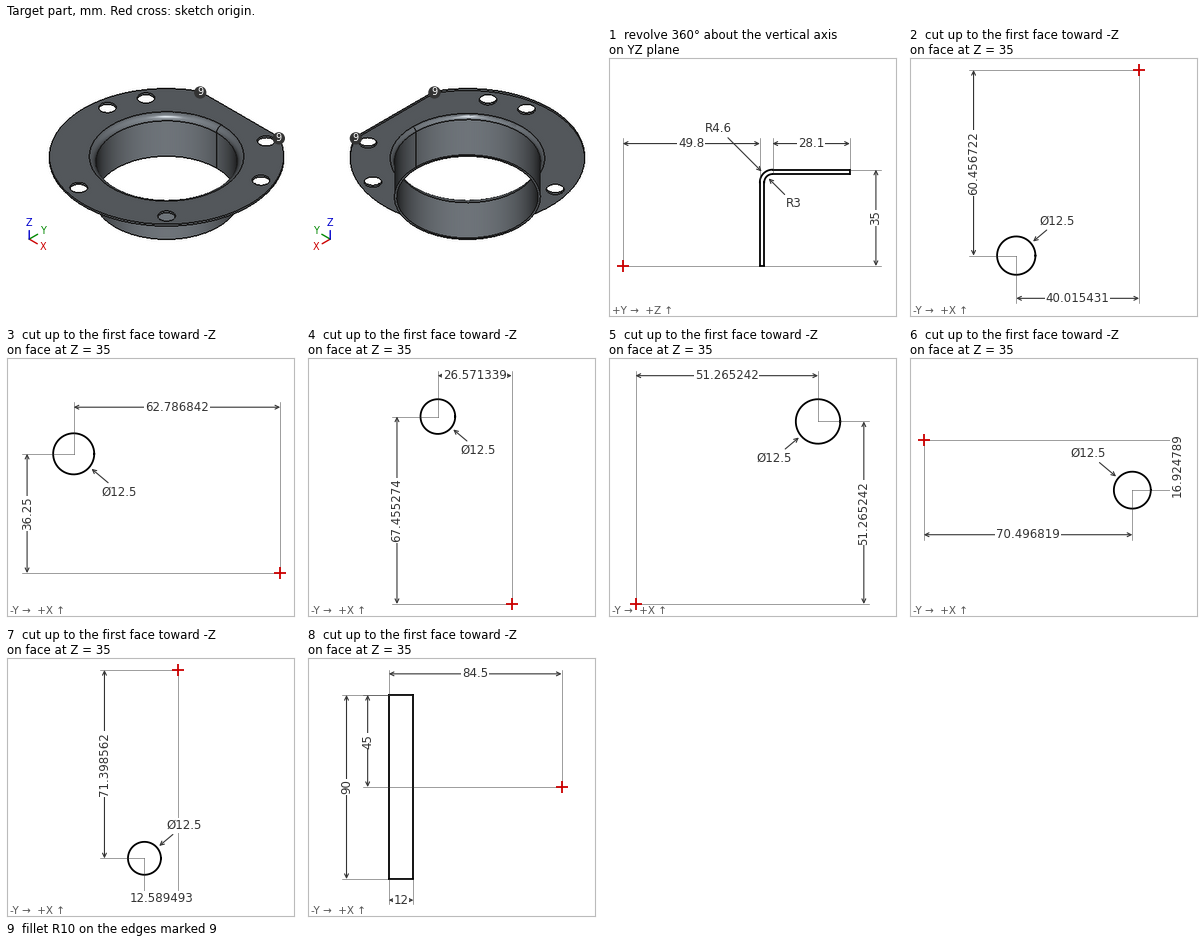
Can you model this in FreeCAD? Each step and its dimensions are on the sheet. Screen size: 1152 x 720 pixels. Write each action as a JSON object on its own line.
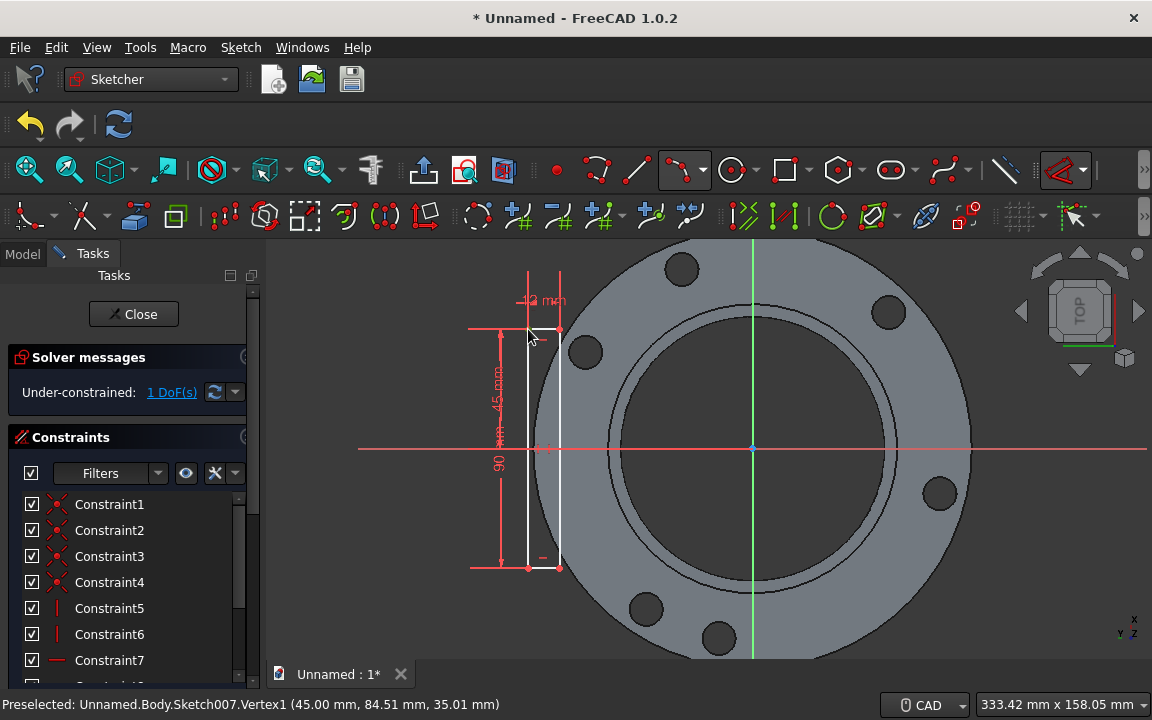
{"action": "key", "text": "l"}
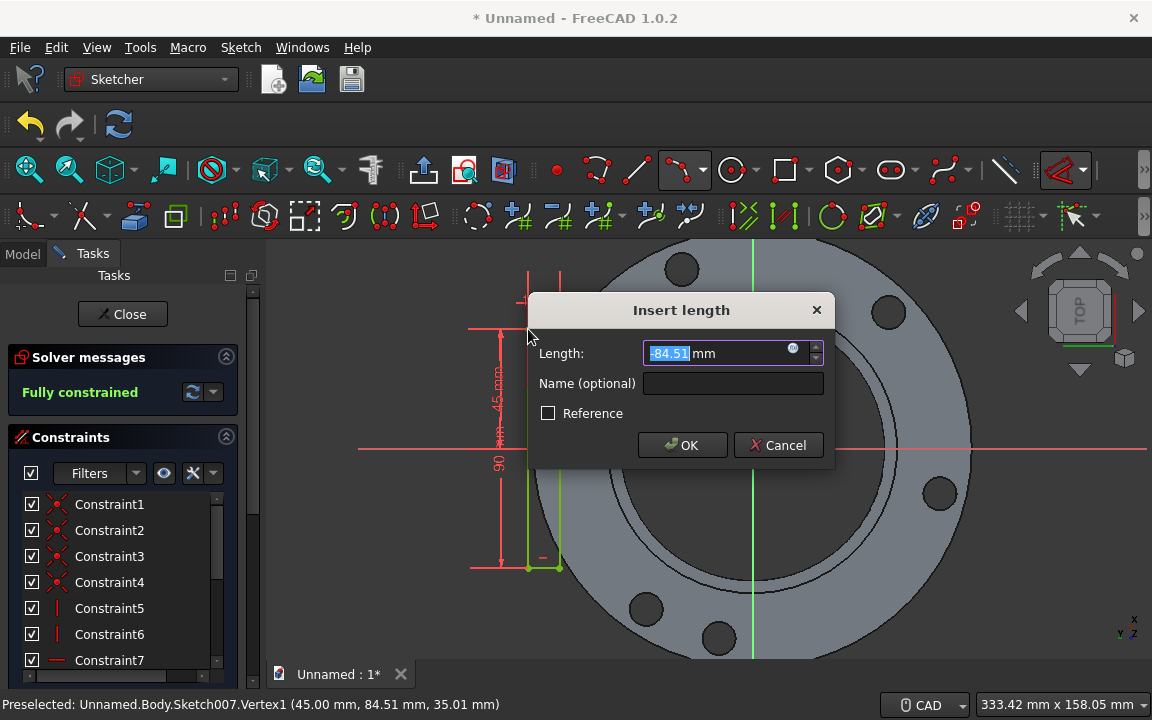
{"action": "type", "text": "-84.5"}
{"action": "key", "text": "Return"}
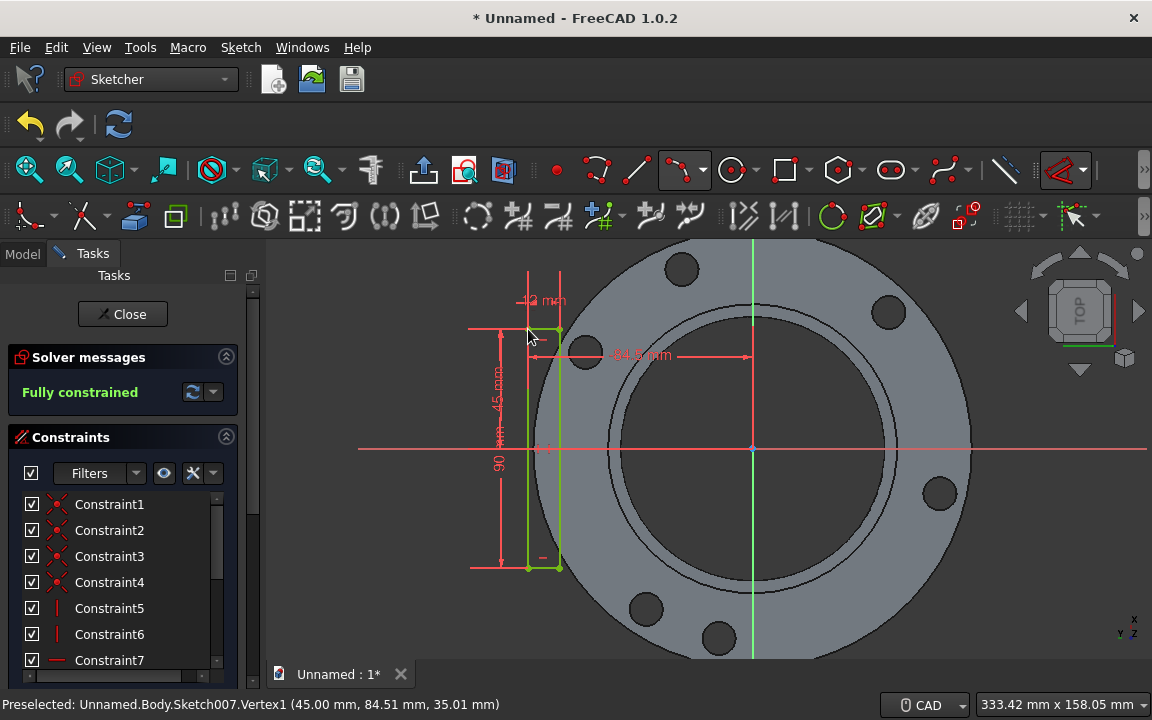
{"action": "left_click", "coordinate": [123, 314]}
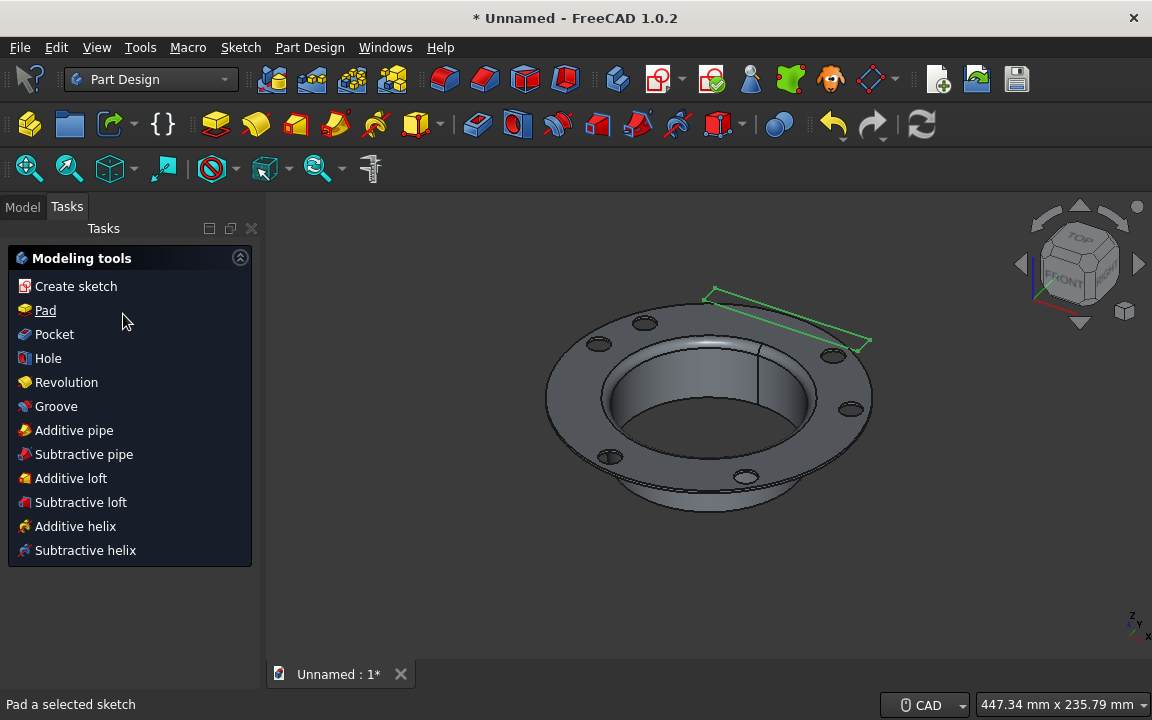
{"action": "left_click", "coordinate": [478, 124]}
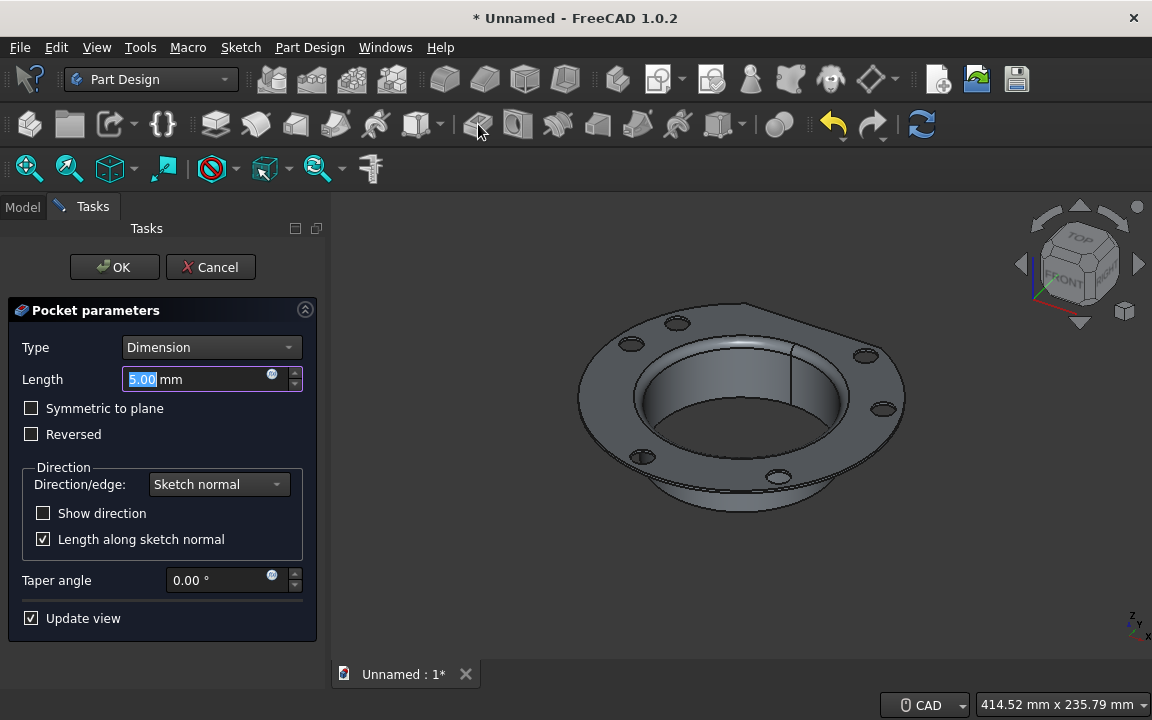
{"action": "left_click", "coordinate": [212, 348]}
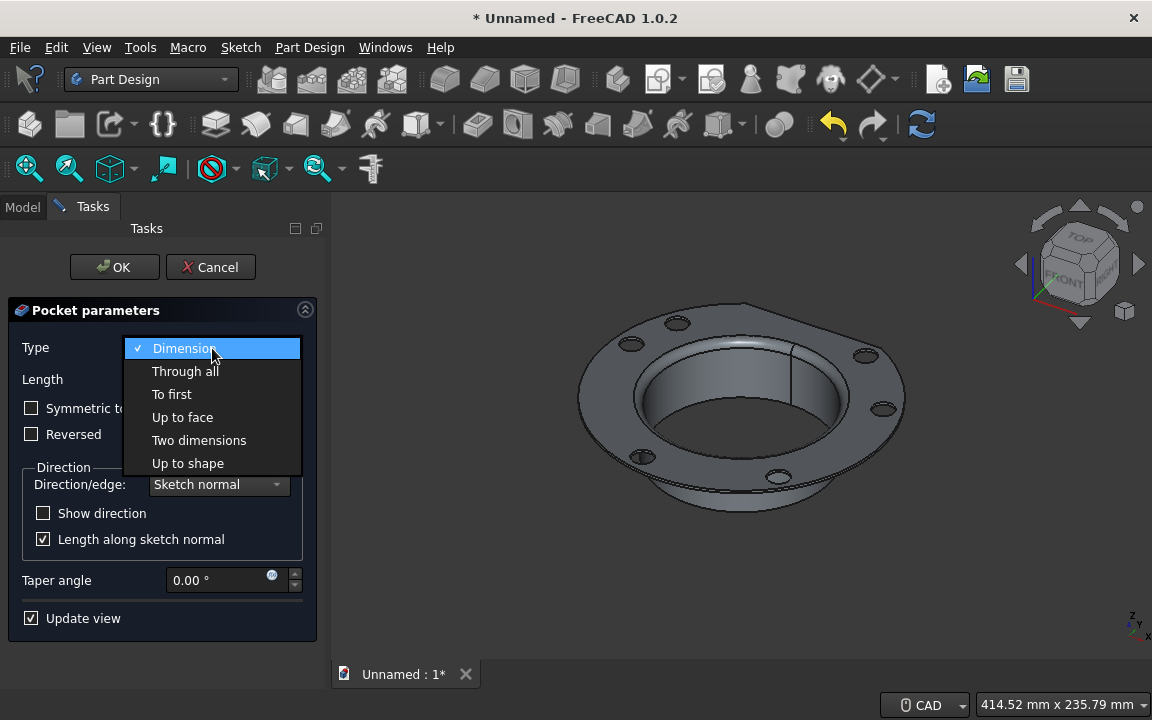
{"action": "left_click", "coordinate": [212, 394]}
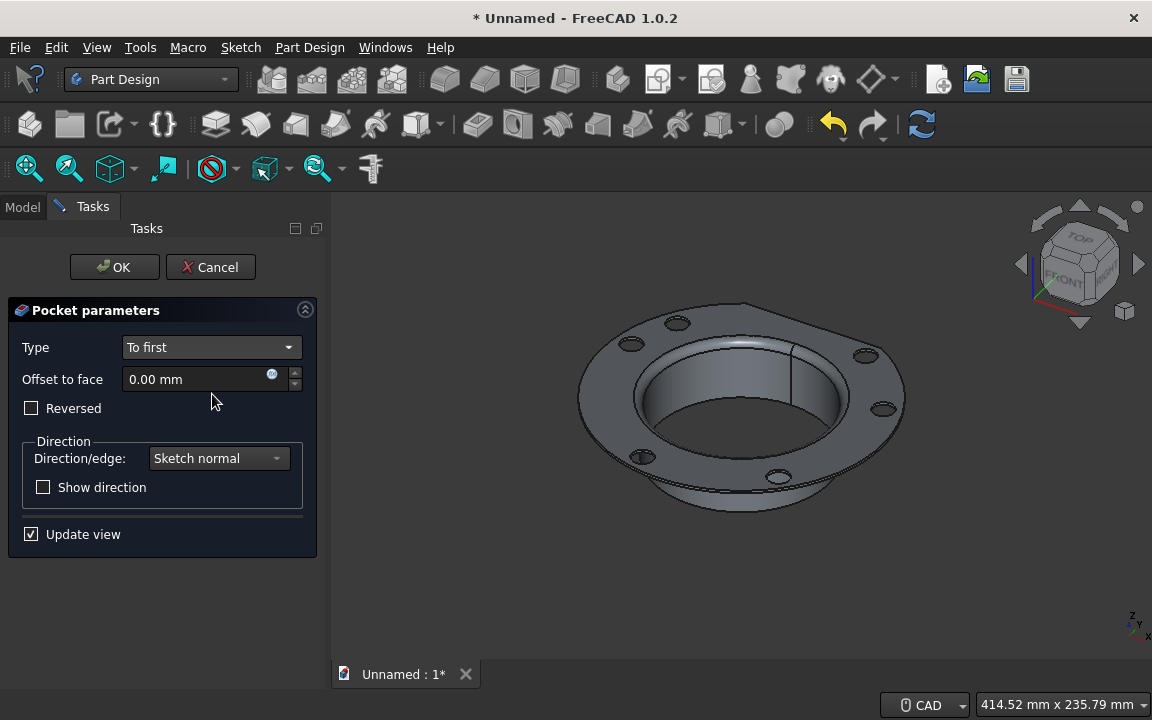
{"action": "left_click", "coordinate": [115, 267]}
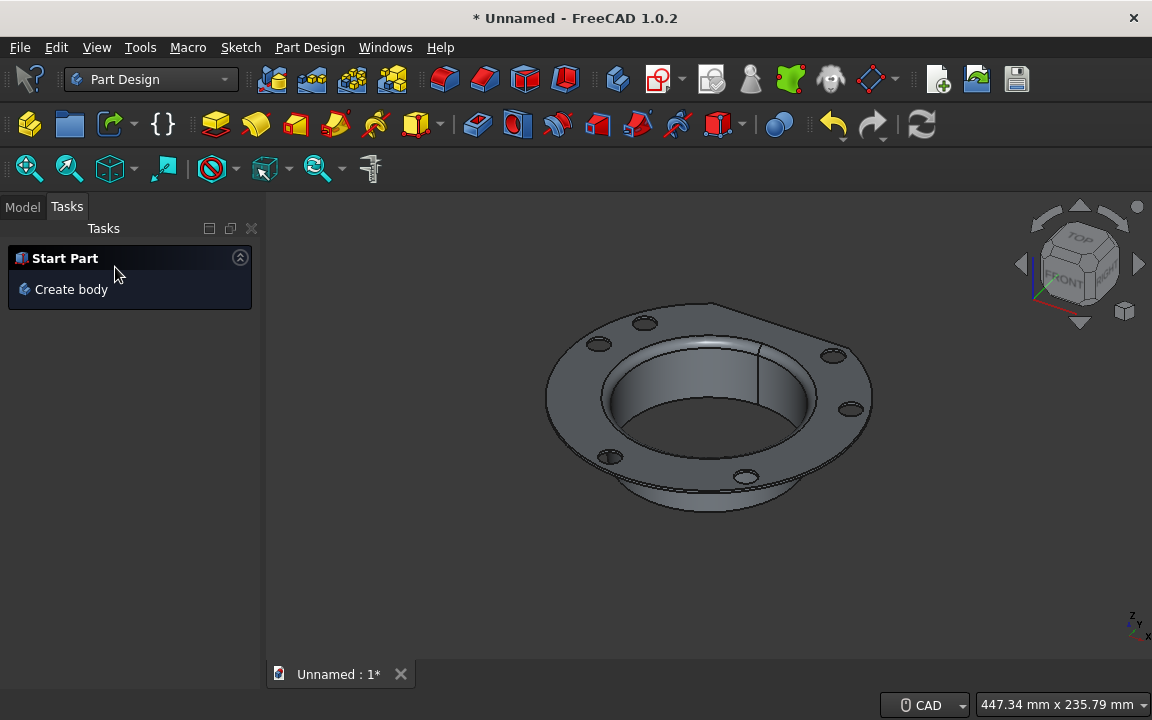
{"action": "scroll", "coordinate": [713, 304], "scroll_direction": "up", "scroll_amount": 13}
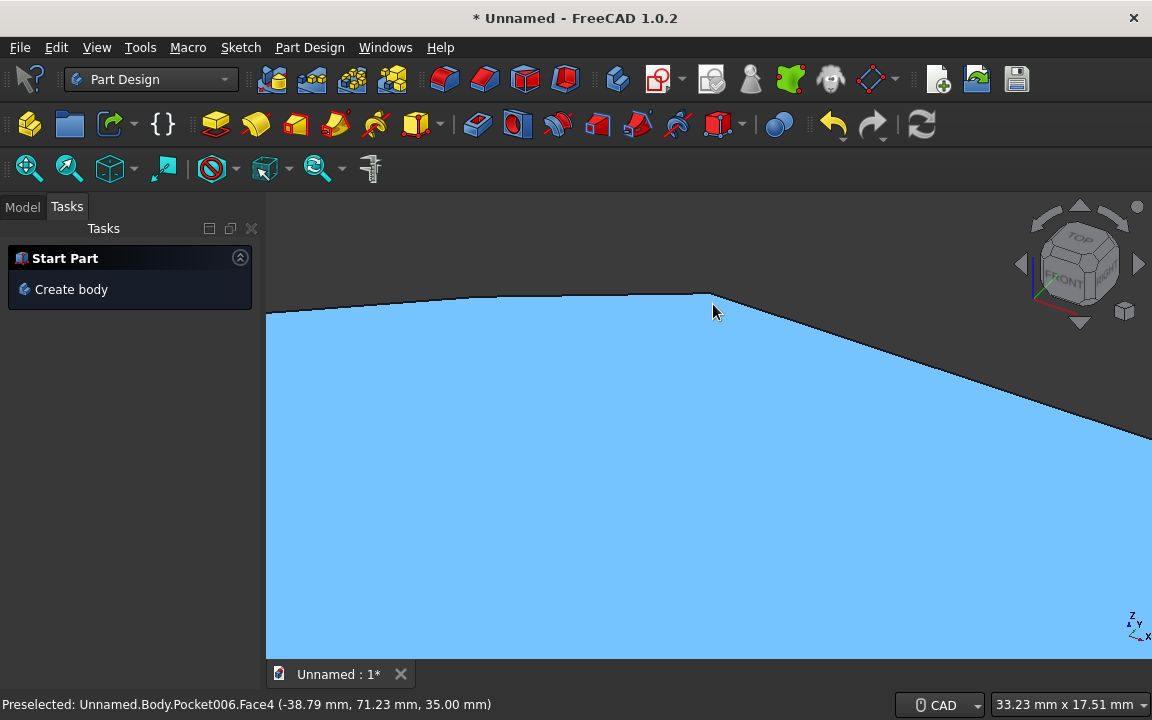
{"action": "left_click", "coordinate": [30, 170]}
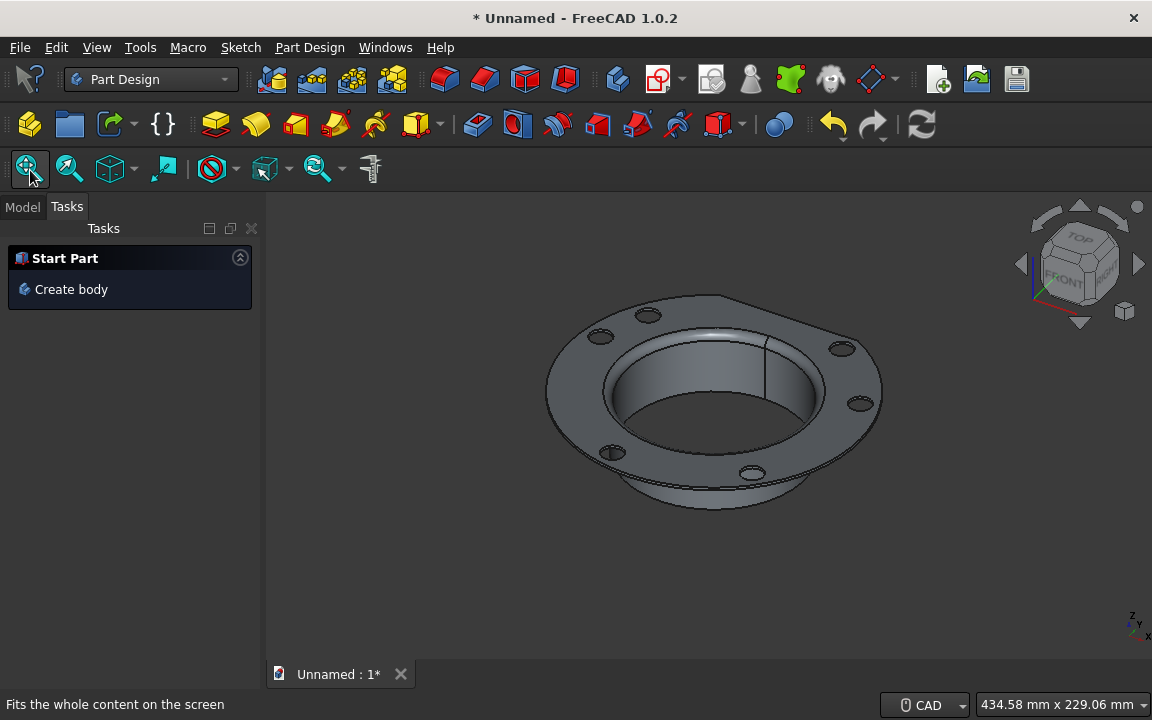
{"action": "key", "text": "0"}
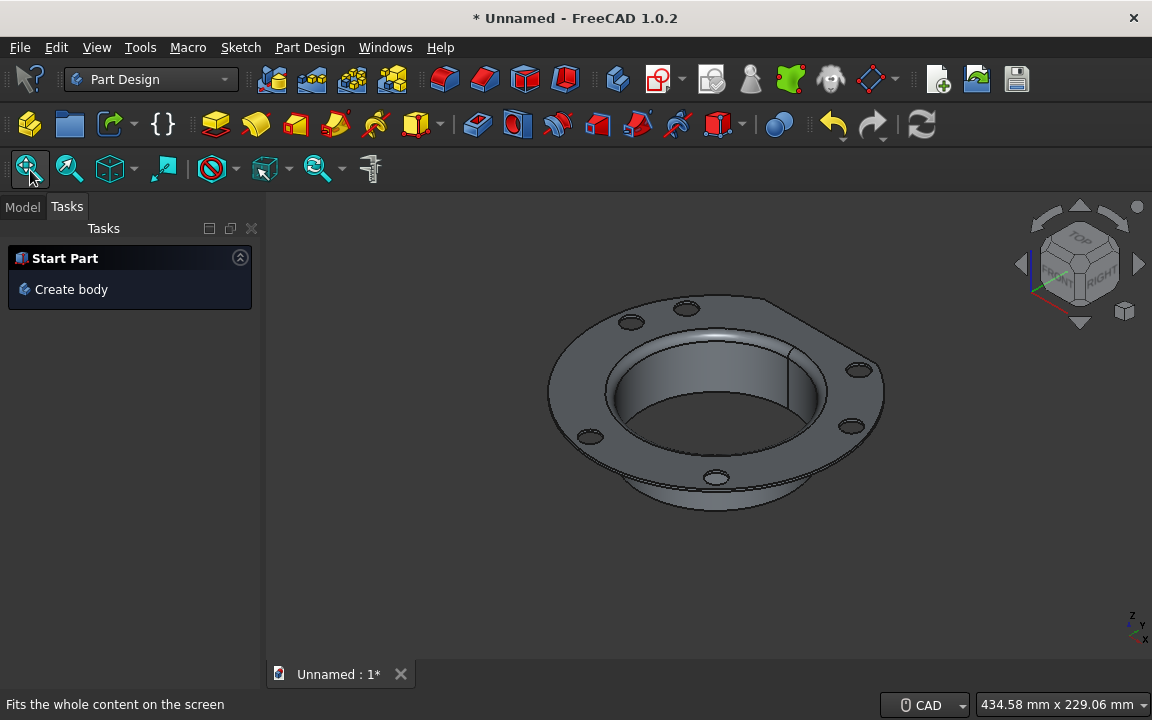
{"action": "scroll", "coordinate": [764, 299], "scroll_direction": "up", "scroll_amount": 13}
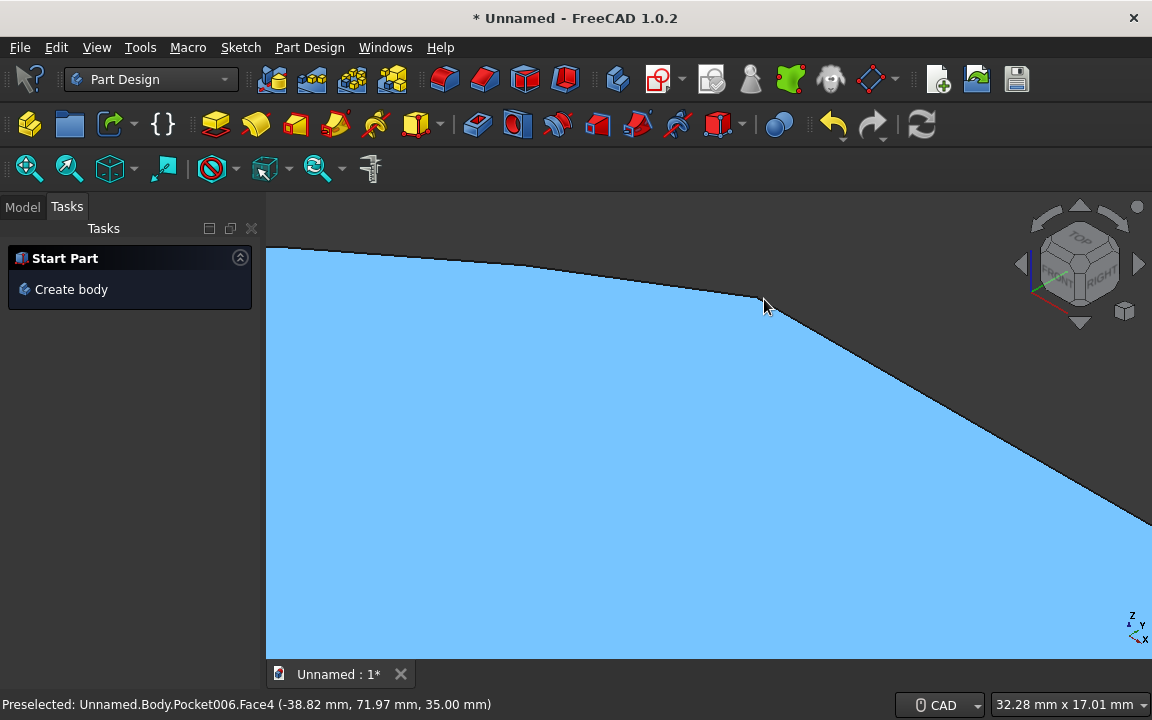
{"action": "key", "text": "v f"}